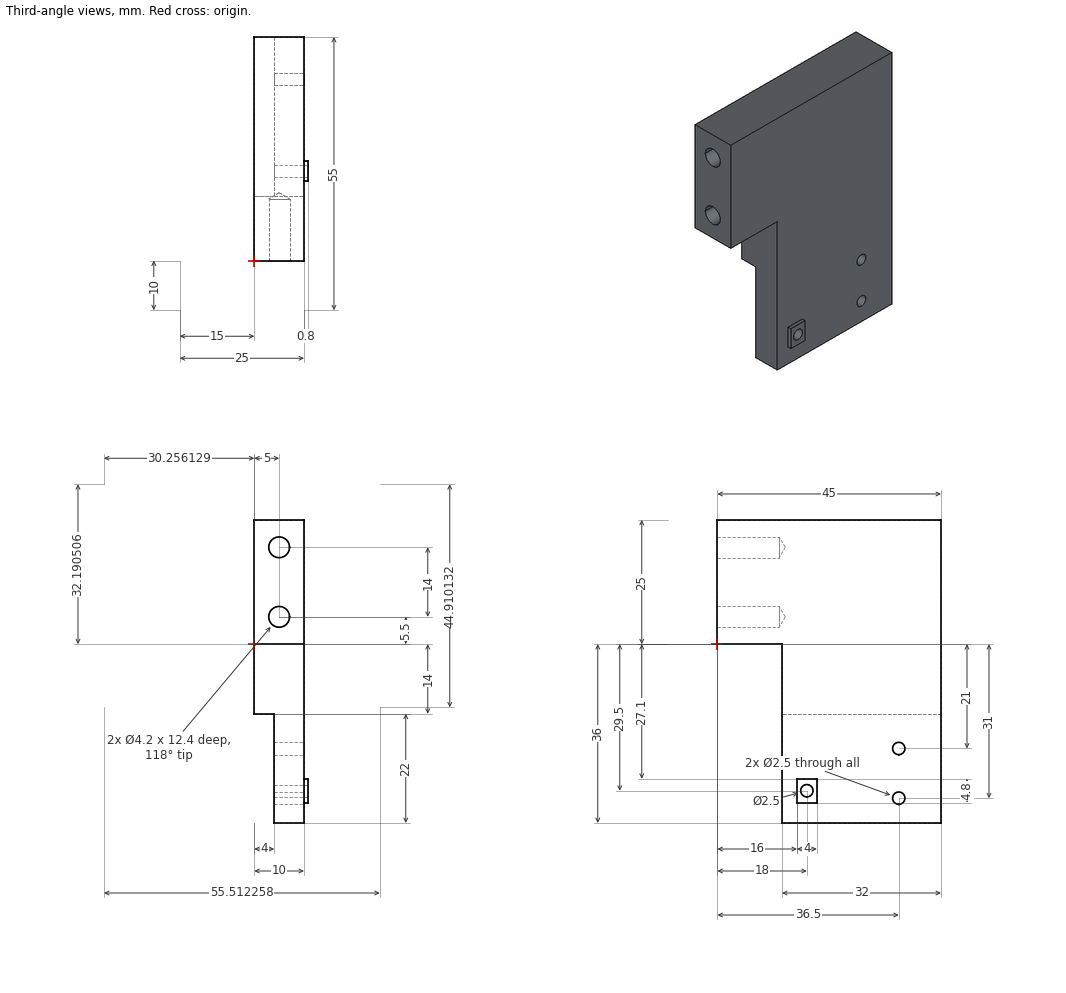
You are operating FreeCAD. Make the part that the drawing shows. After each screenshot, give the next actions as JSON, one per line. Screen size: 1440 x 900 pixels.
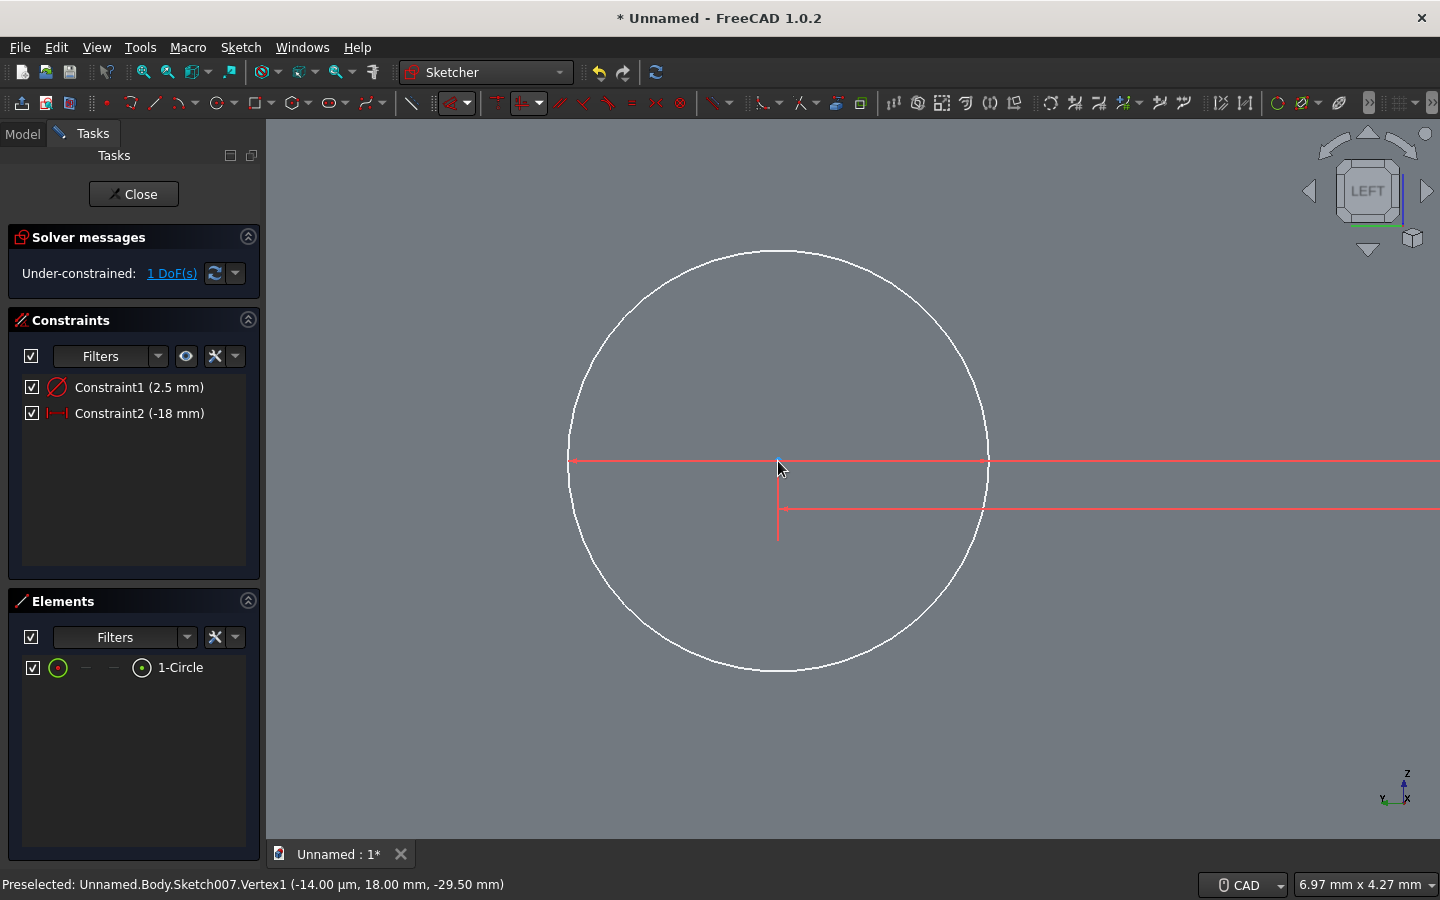
{"action": "left_click", "coordinate": [778, 461]}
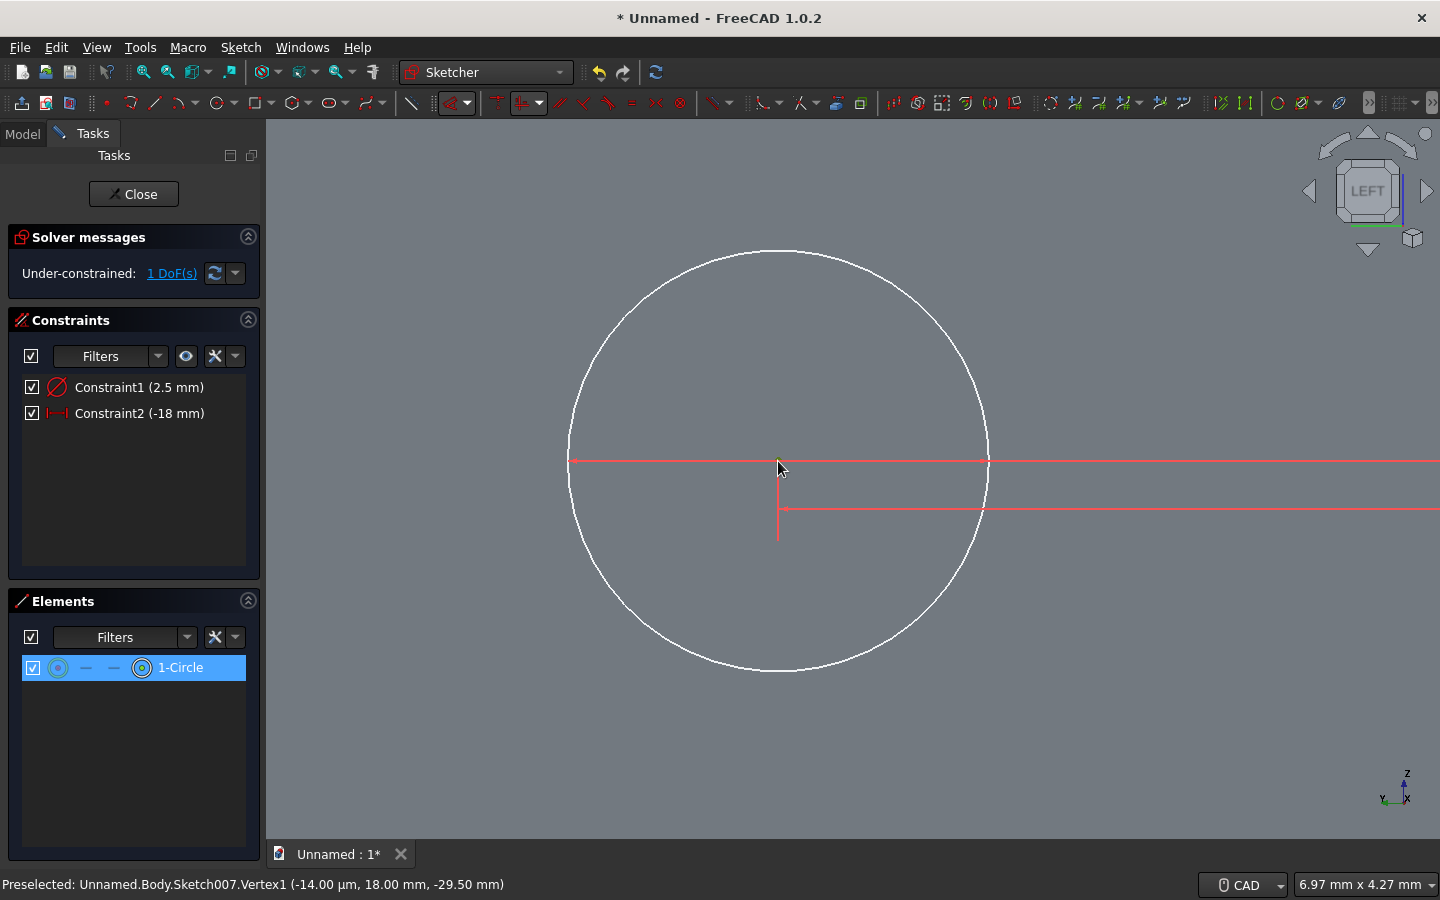
{"action": "left_click", "coordinate": [470, 104]}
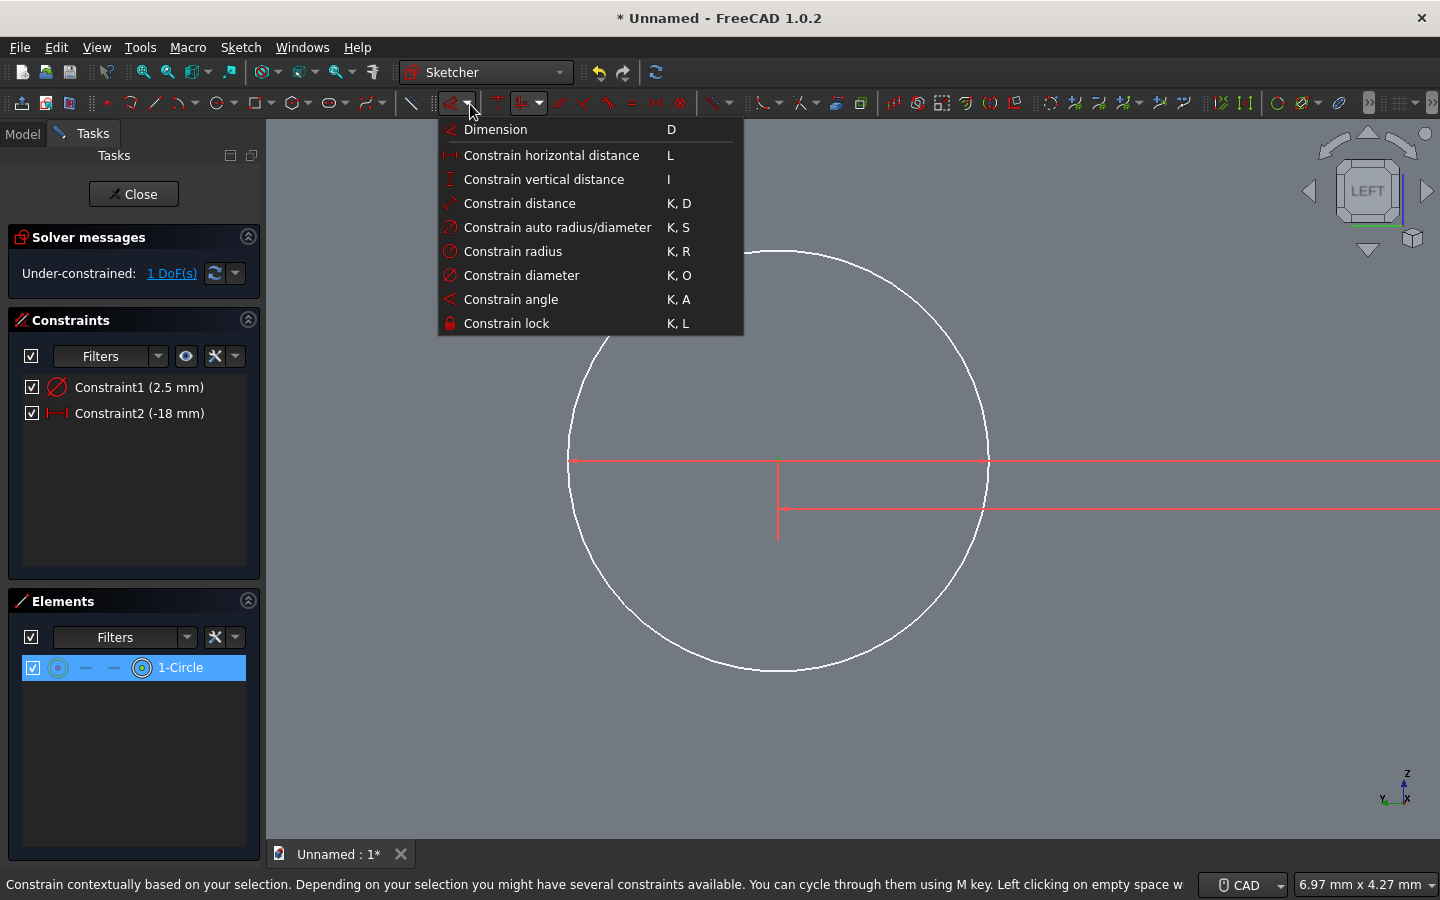
{"action": "left_click", "coordinate": [591, 179]}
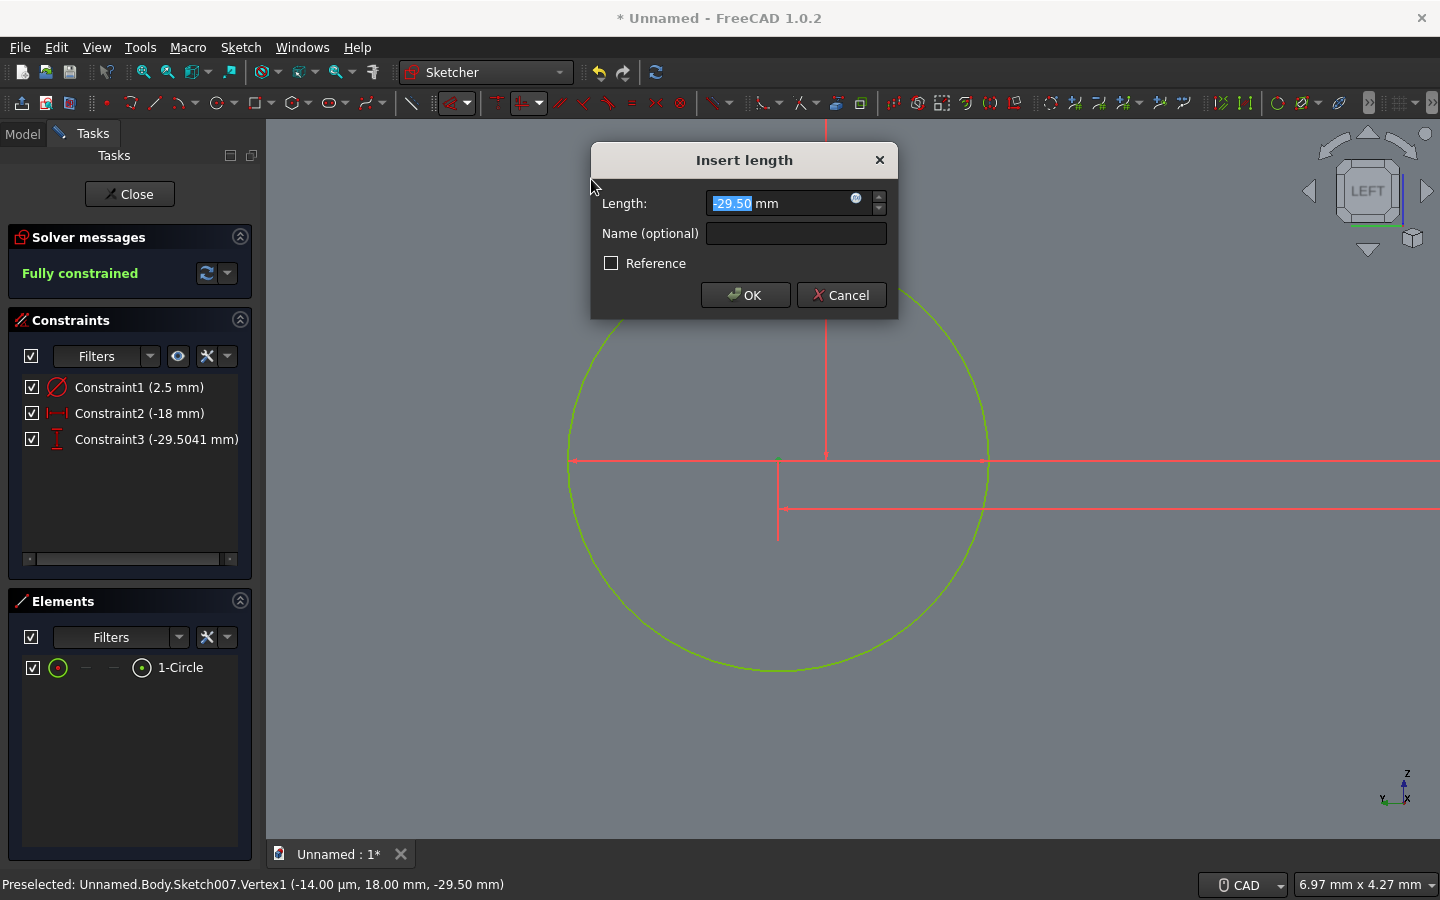
{"action": "type", "text": "-29.5"}
{"action": "key", "text": "Return"}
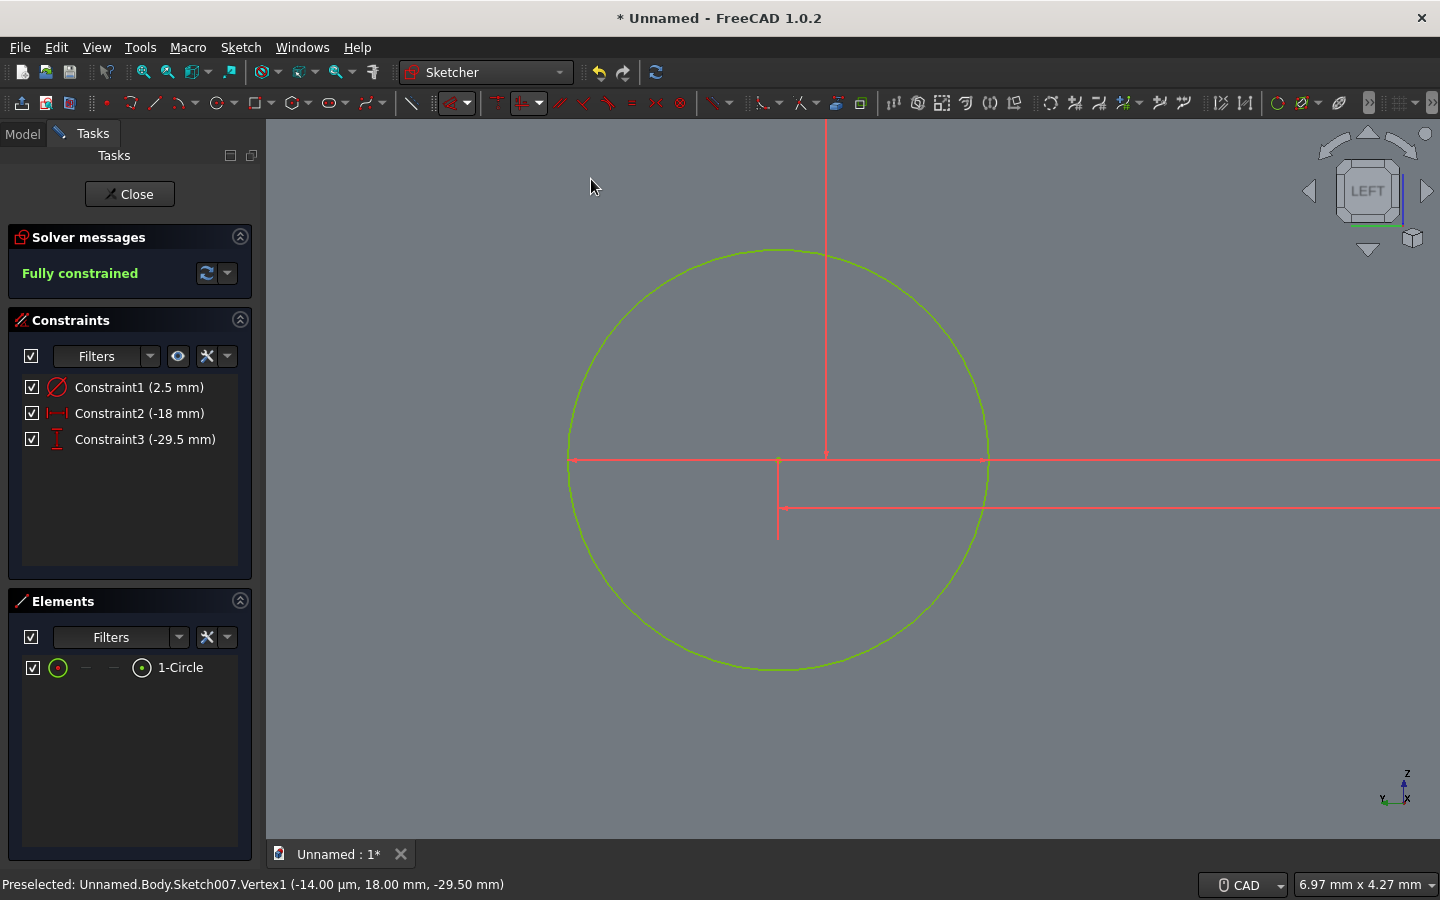
{"action": "left_click", "coordinate": [130, 194]}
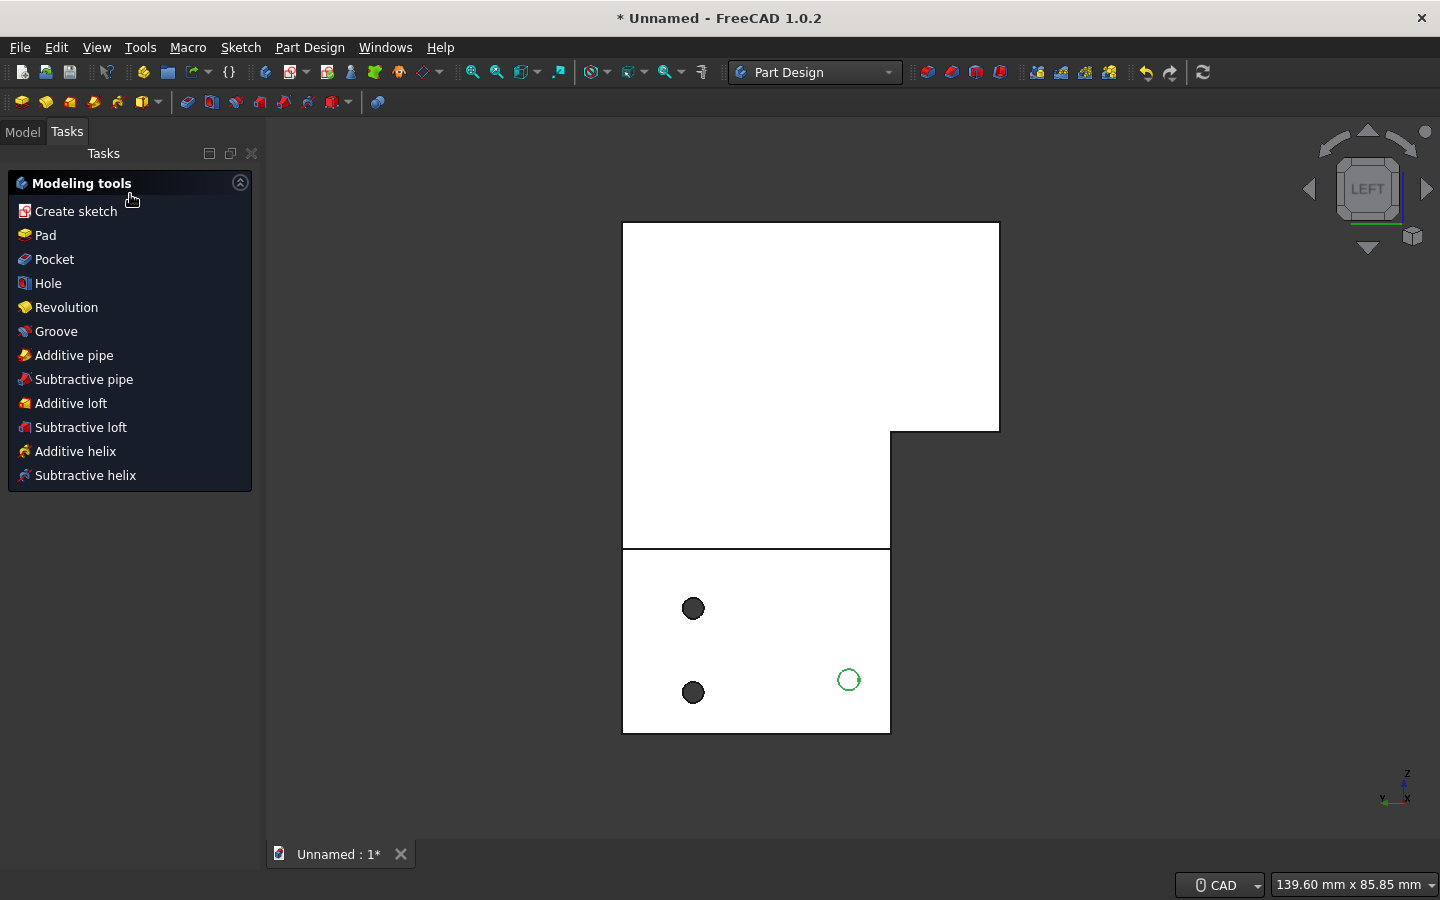
{"action": "left_click", "coordinate": [188, 102]}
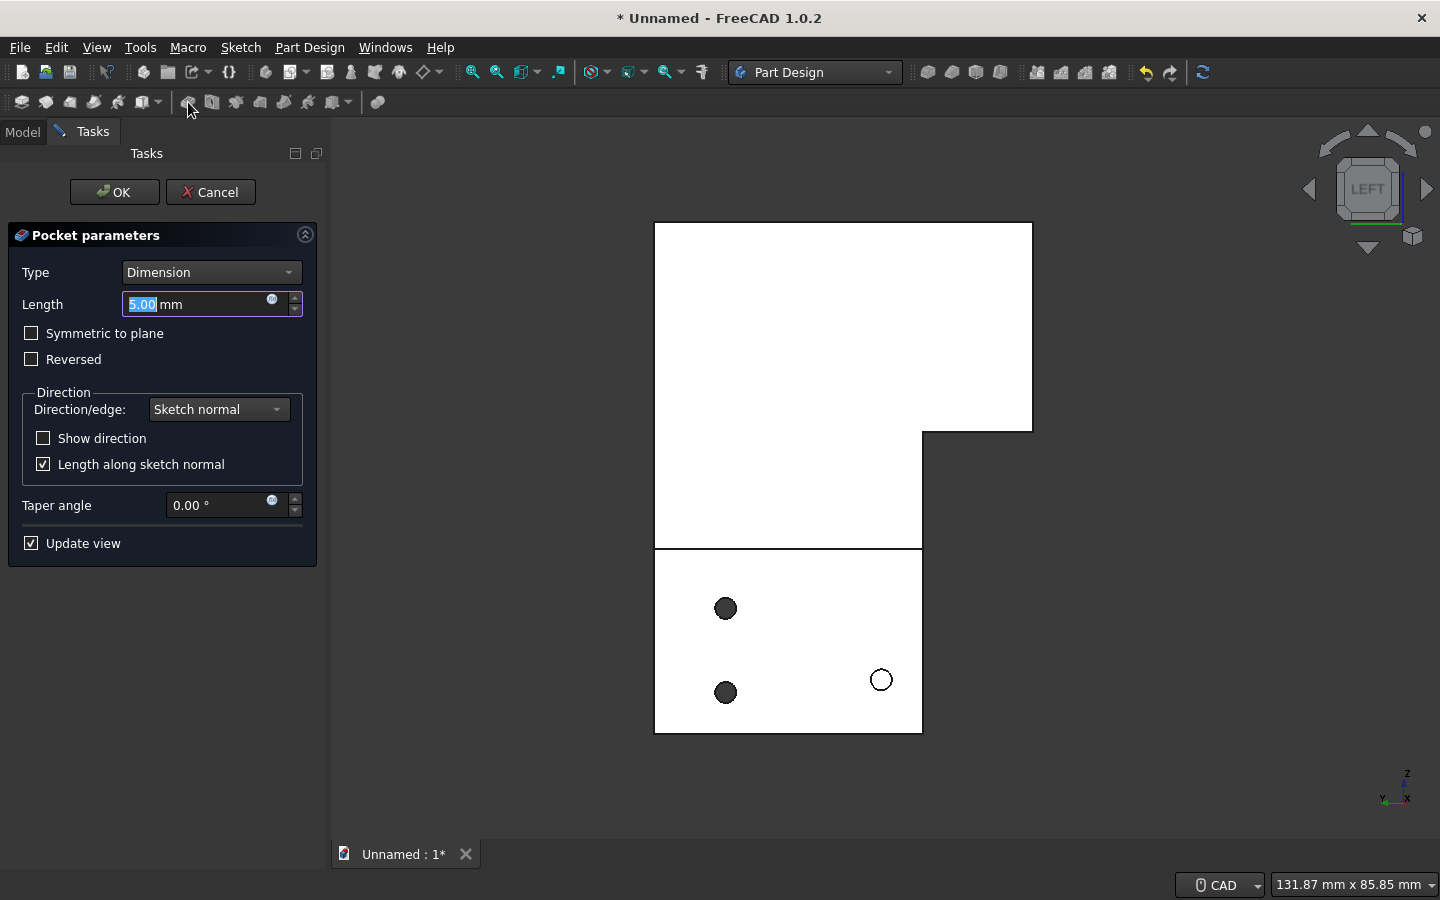
{"action": "left_click", "coordinate": [212, 272]}